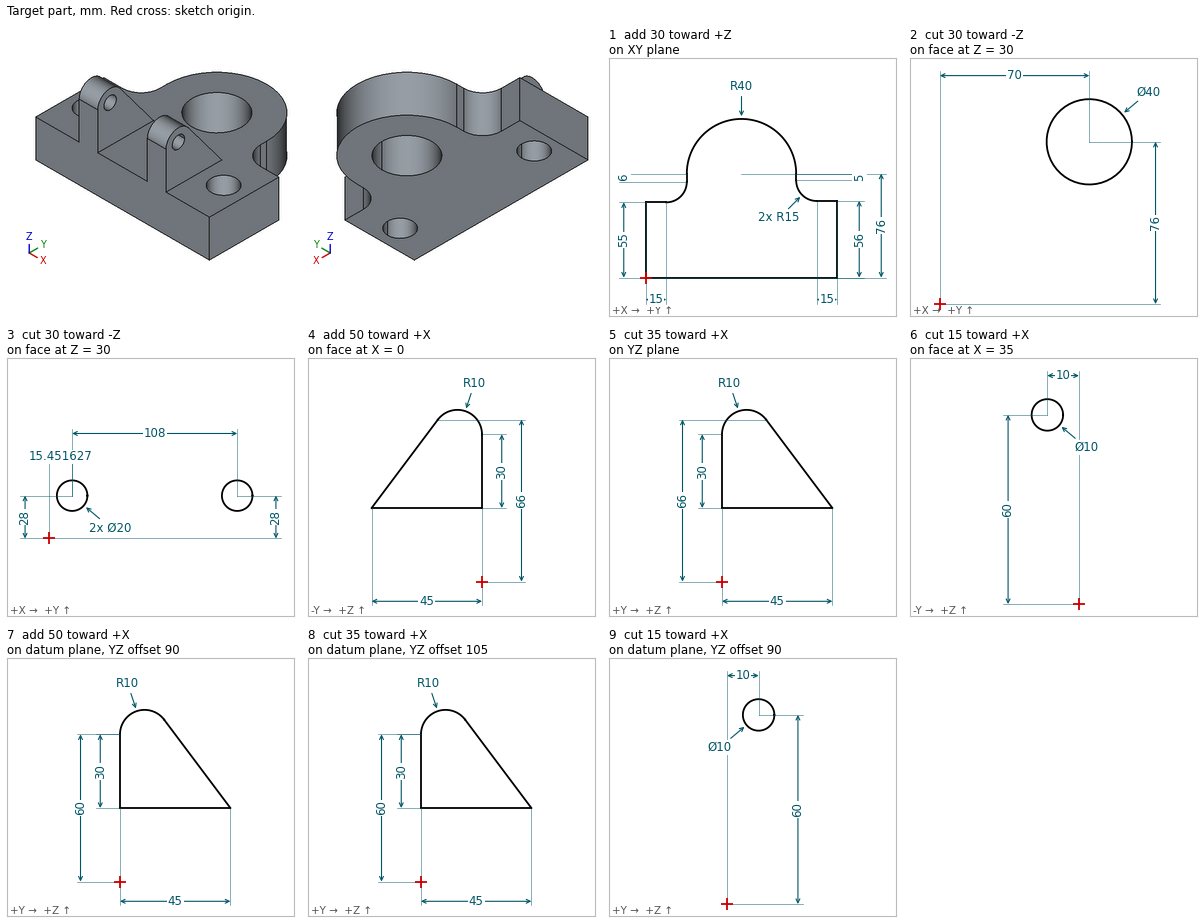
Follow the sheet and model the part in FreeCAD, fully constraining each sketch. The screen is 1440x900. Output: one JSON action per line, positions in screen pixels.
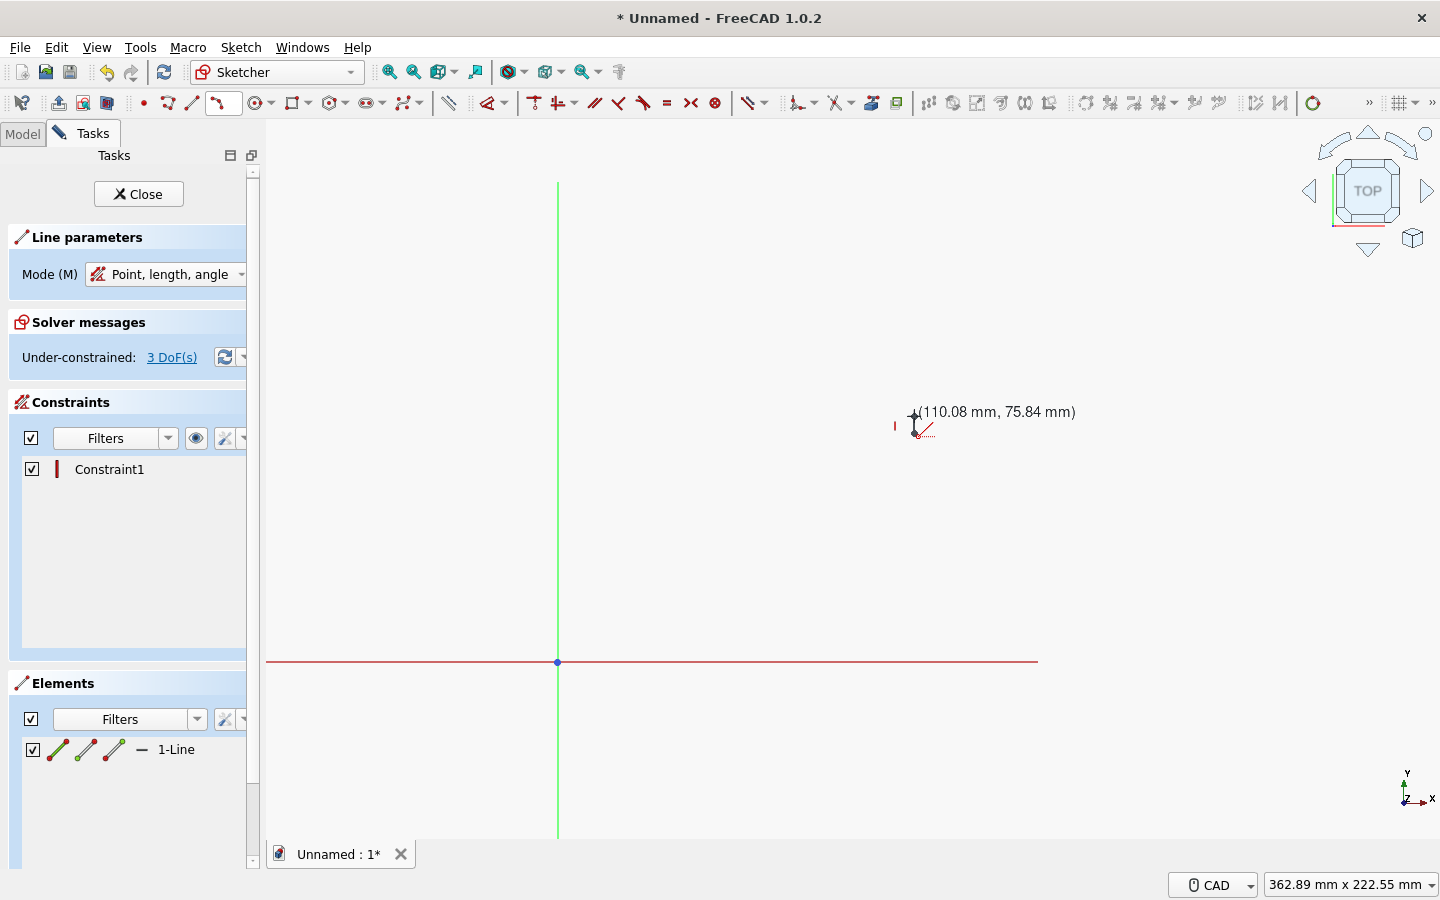
{"action": "left_click", "coordinate": [655, 416]}
{"action": "left_click", "coordinate": [655, 436]}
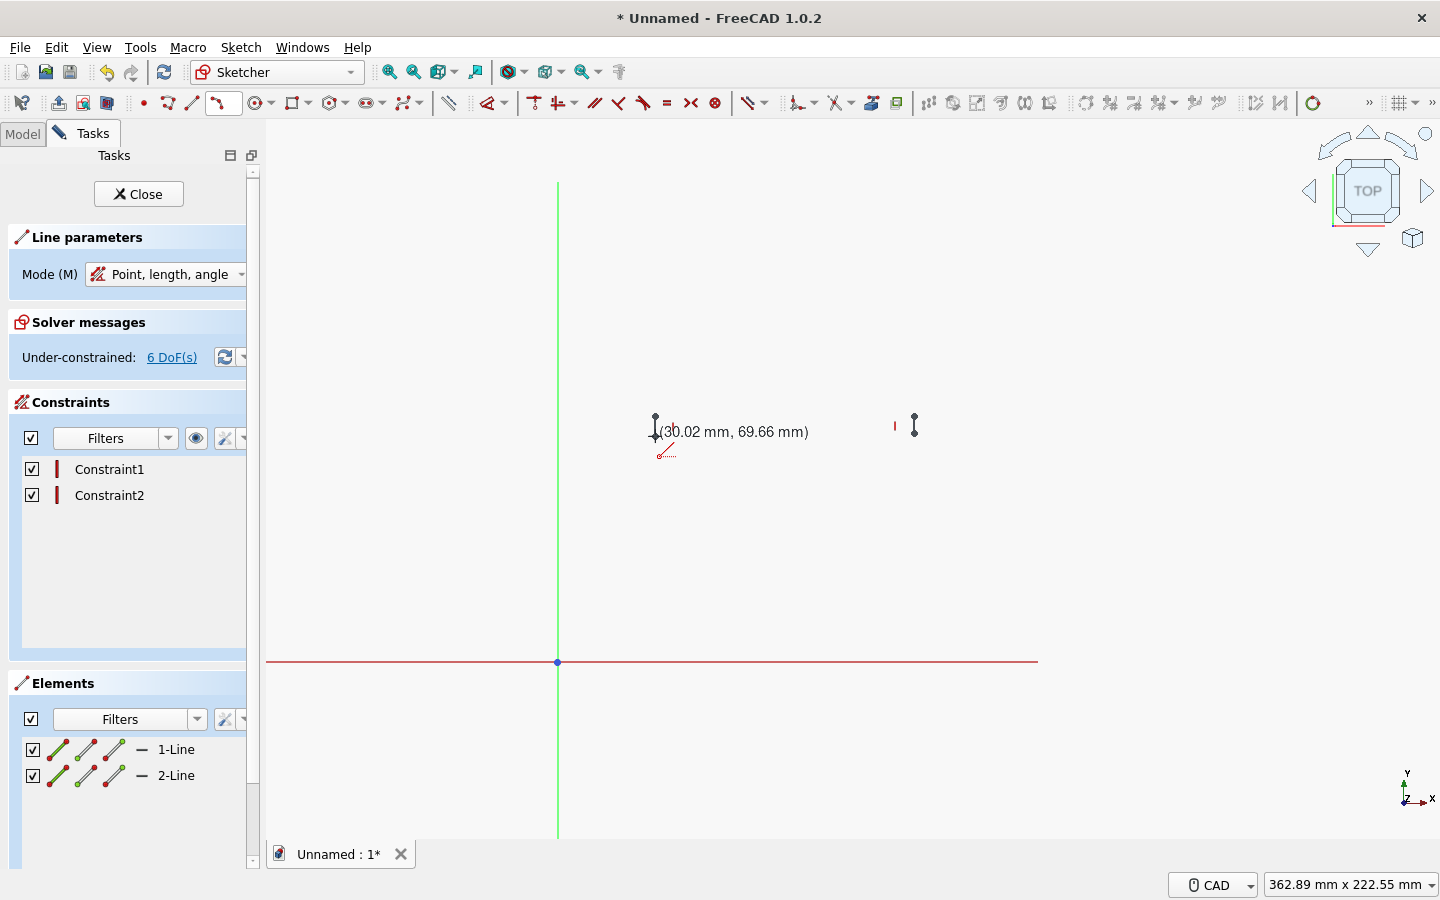
{"action": "key", "text": "g m"}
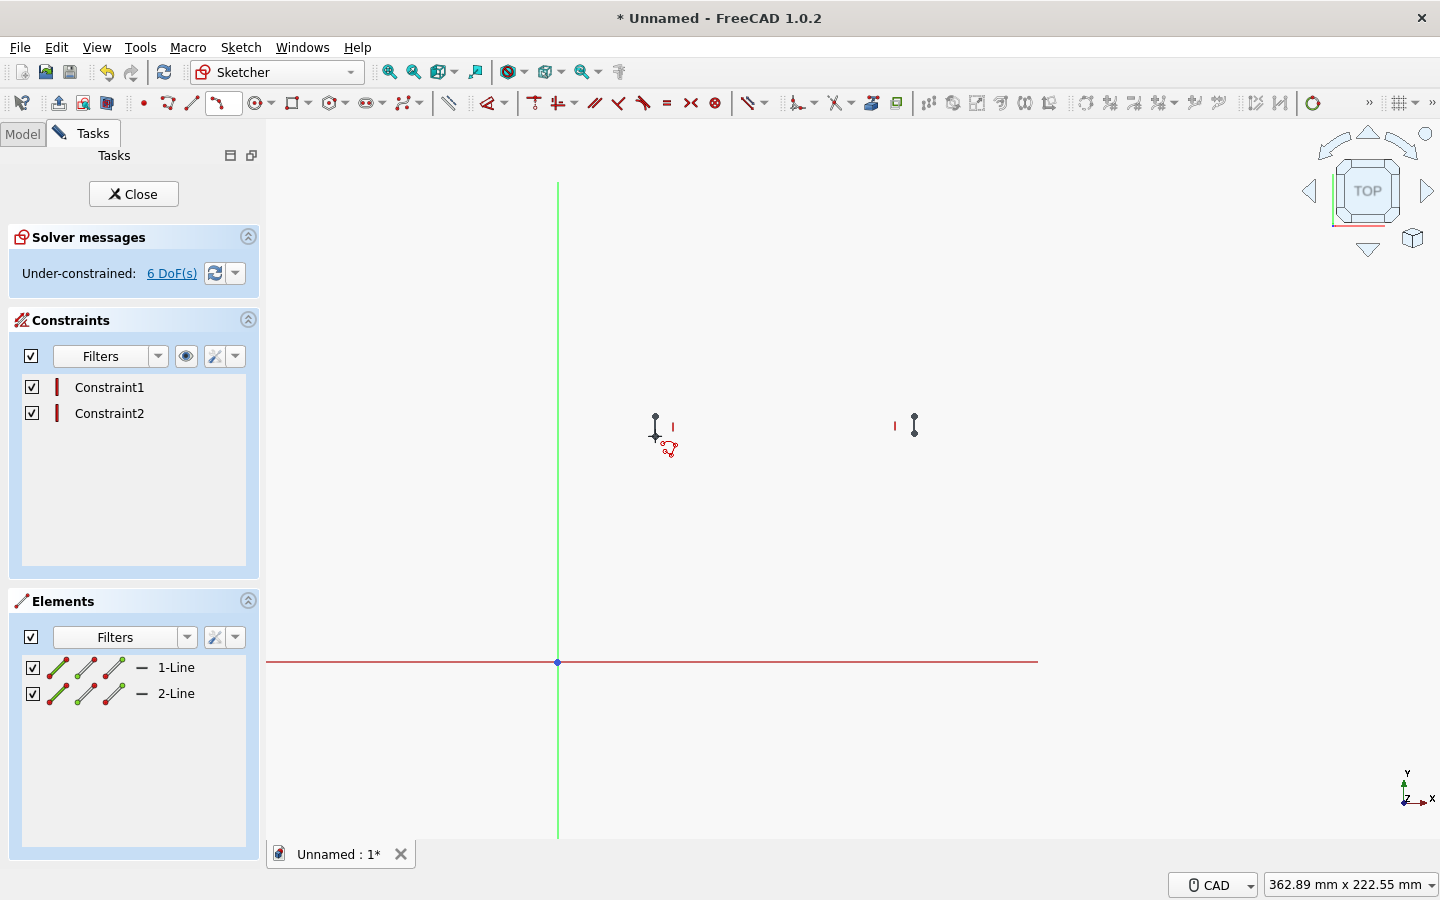
{"action": "left_click", "coordinate": [606, 484]}
{"action": "left_click", "coordinate": [558, 484]}
{"action": "left_click", "coordinate": [558, 662]}
{"action": "left_click", "coordinate": [1011, 653]}
{"action": "left_click", "coordinate": [1011, 481]}
{"action": "left_click", "coordinate": [962, 481]}
{"action": "right_click", "coordinate": [962, 481]}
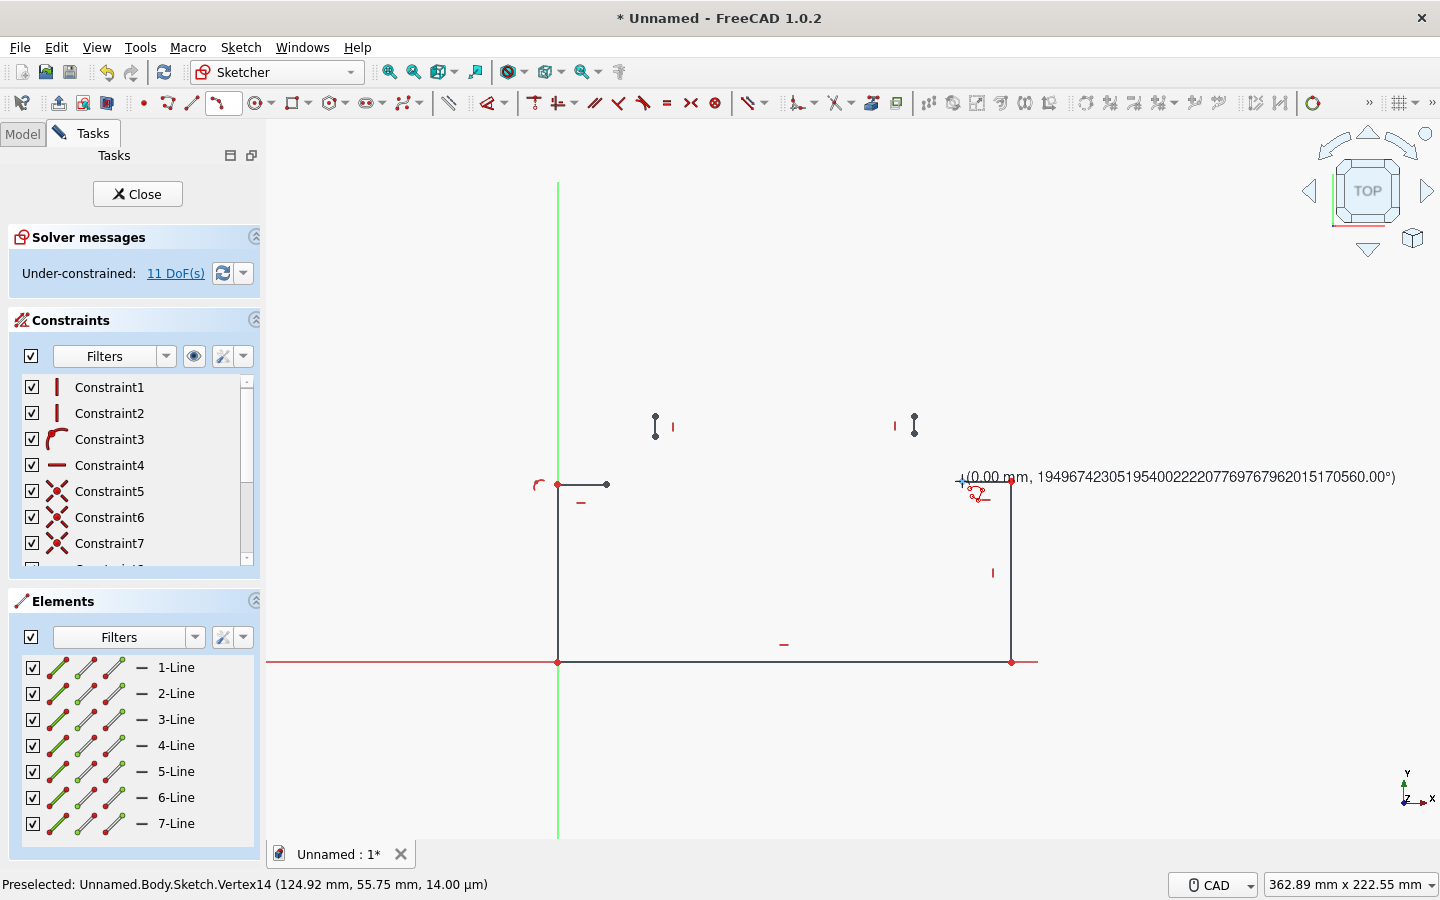
{"action": "left_click", "coordinate": [218, 104]}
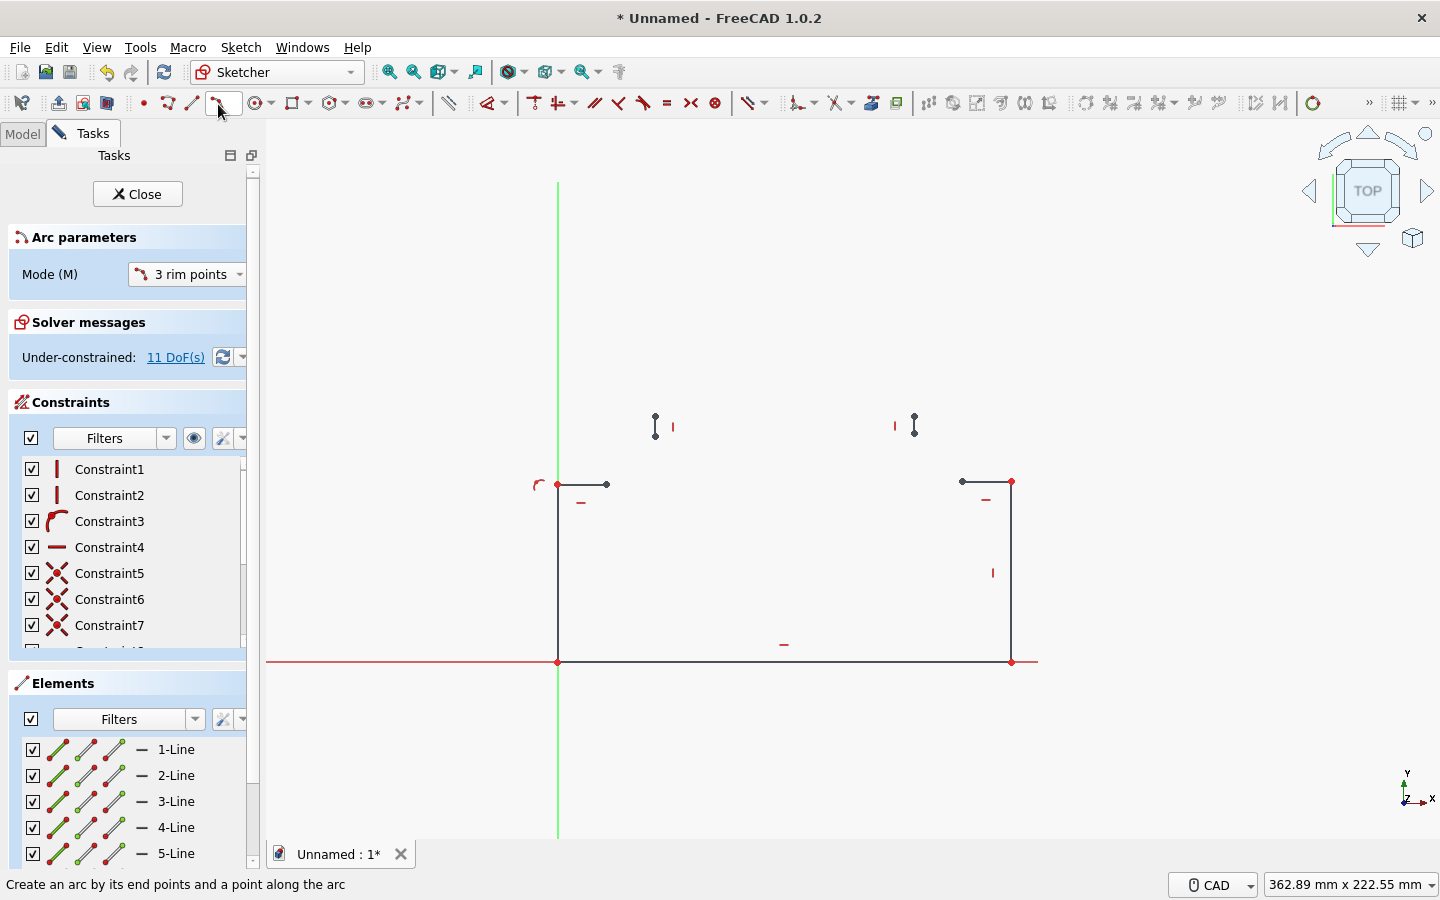
{"action": "scroll", "coordinate": [914, 416], "scroll_direction": "up", "scroll_amount": 4}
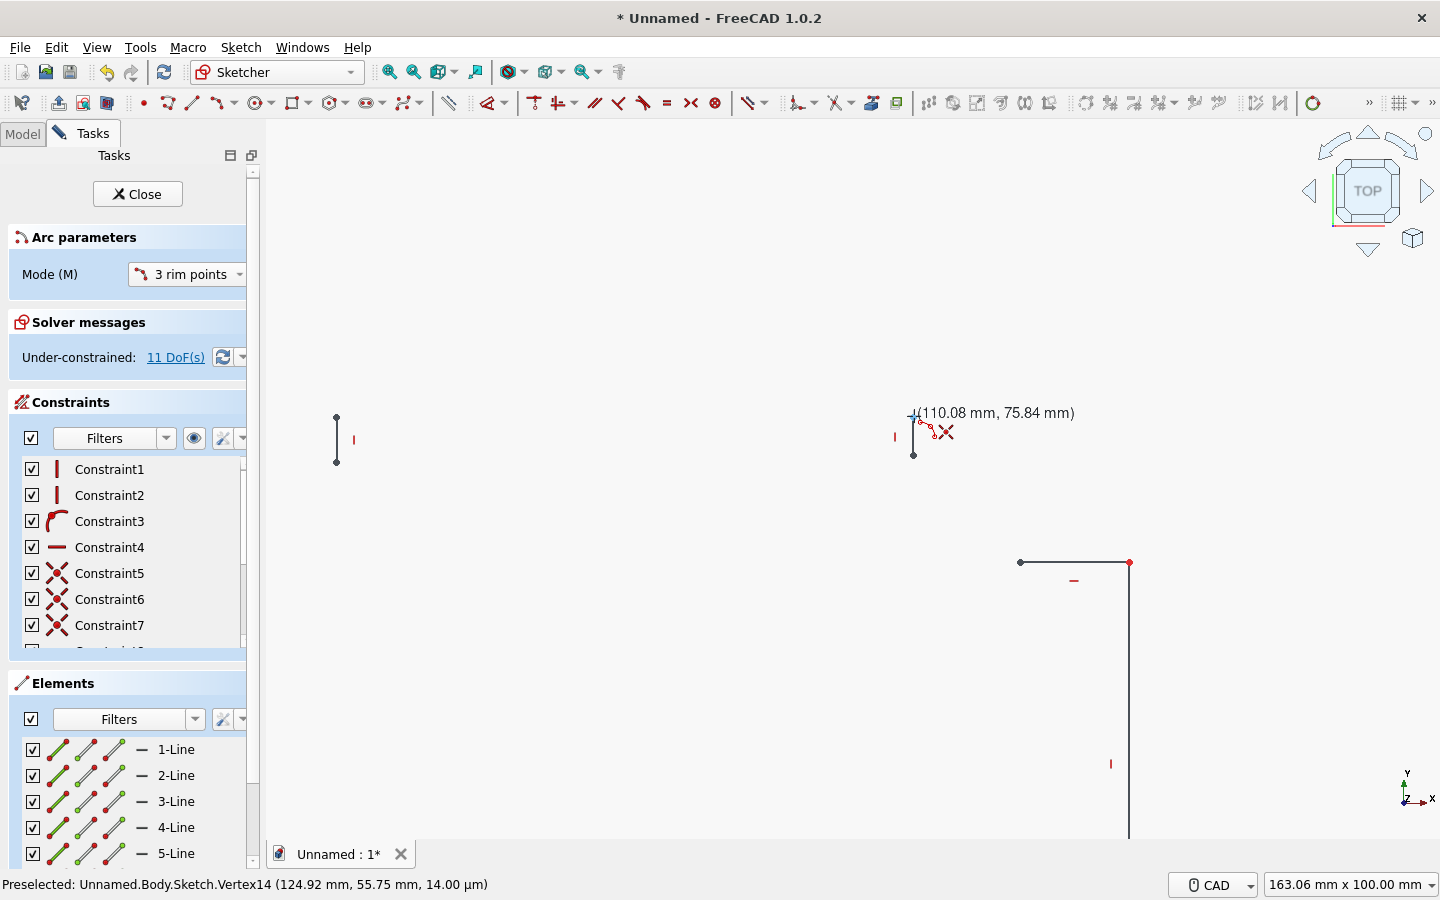
{"action": "left_click", "coordinate": [913, 418]}
{"action": "left_click", "coordinate": [337, 418]}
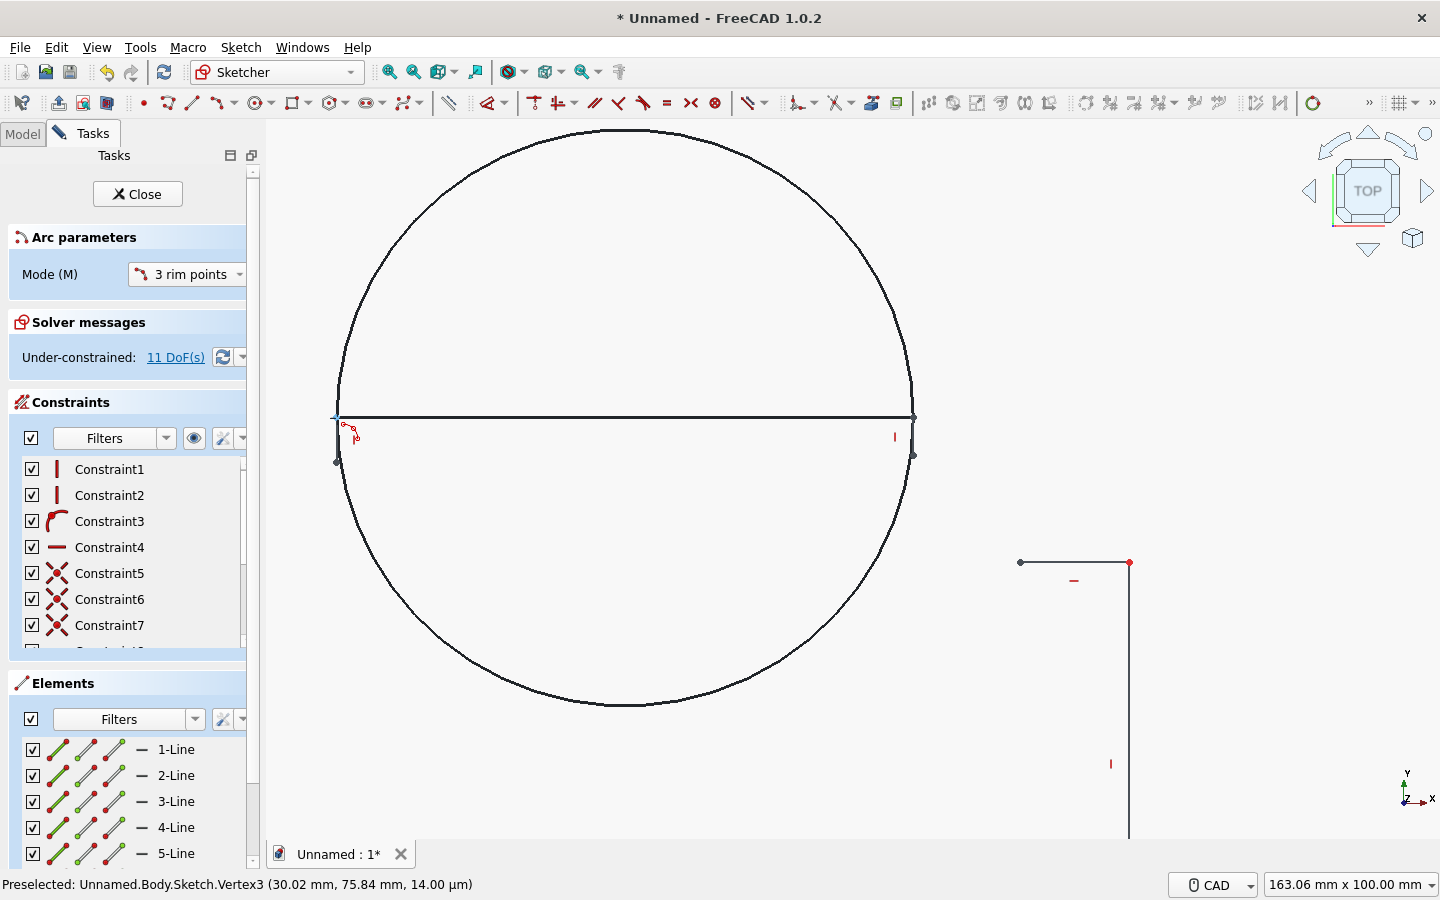
{"action": "scroll", "coordinate": [979, 397], "scroll_direction": "down", "scroll_amount": 3}